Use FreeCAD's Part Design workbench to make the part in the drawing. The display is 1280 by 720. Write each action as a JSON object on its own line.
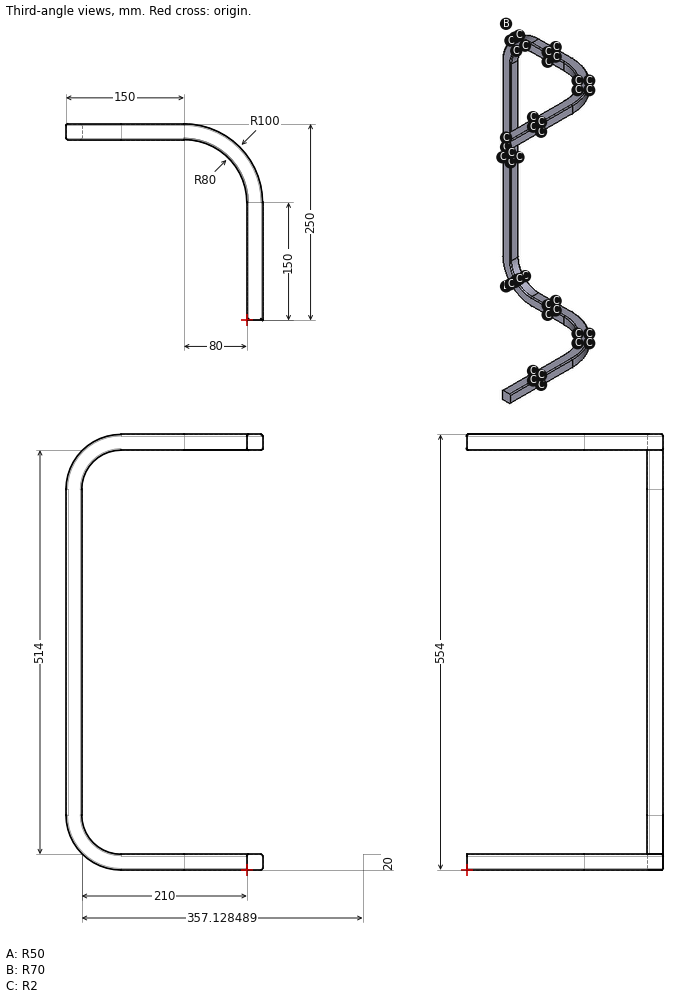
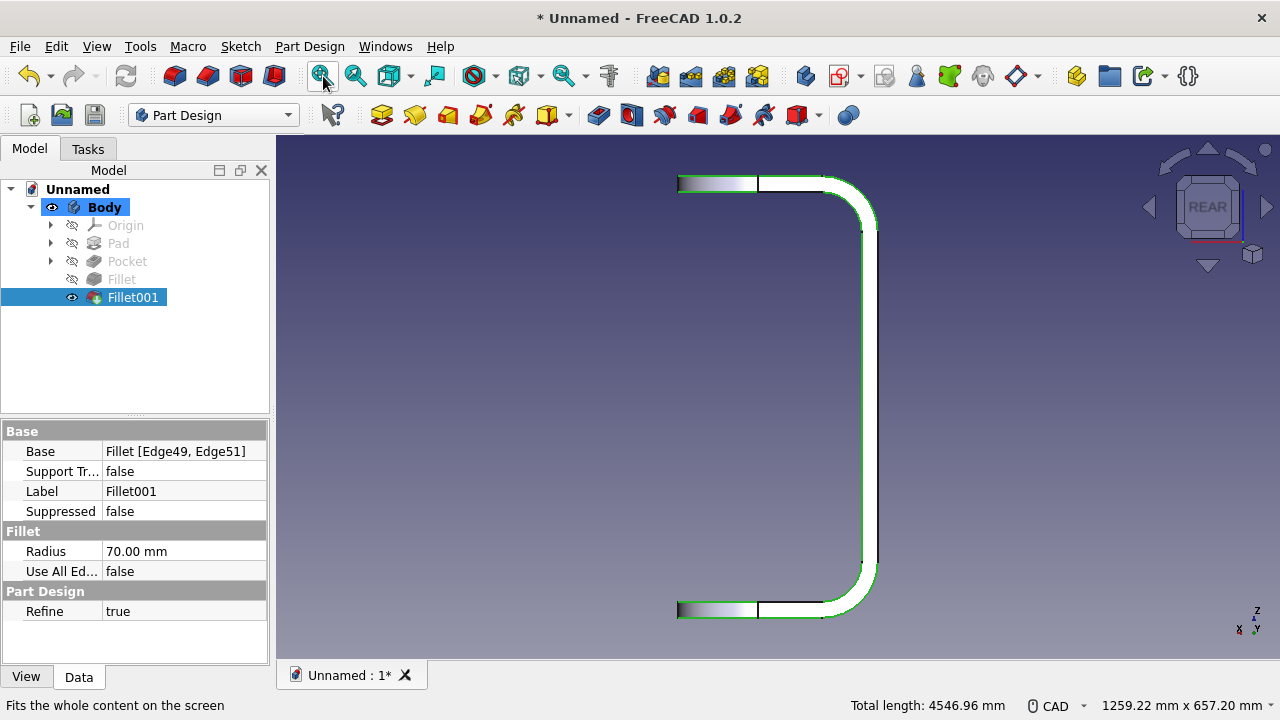
{"action": "left_click", "coordinate": [790, 601], "text": "ctrl"}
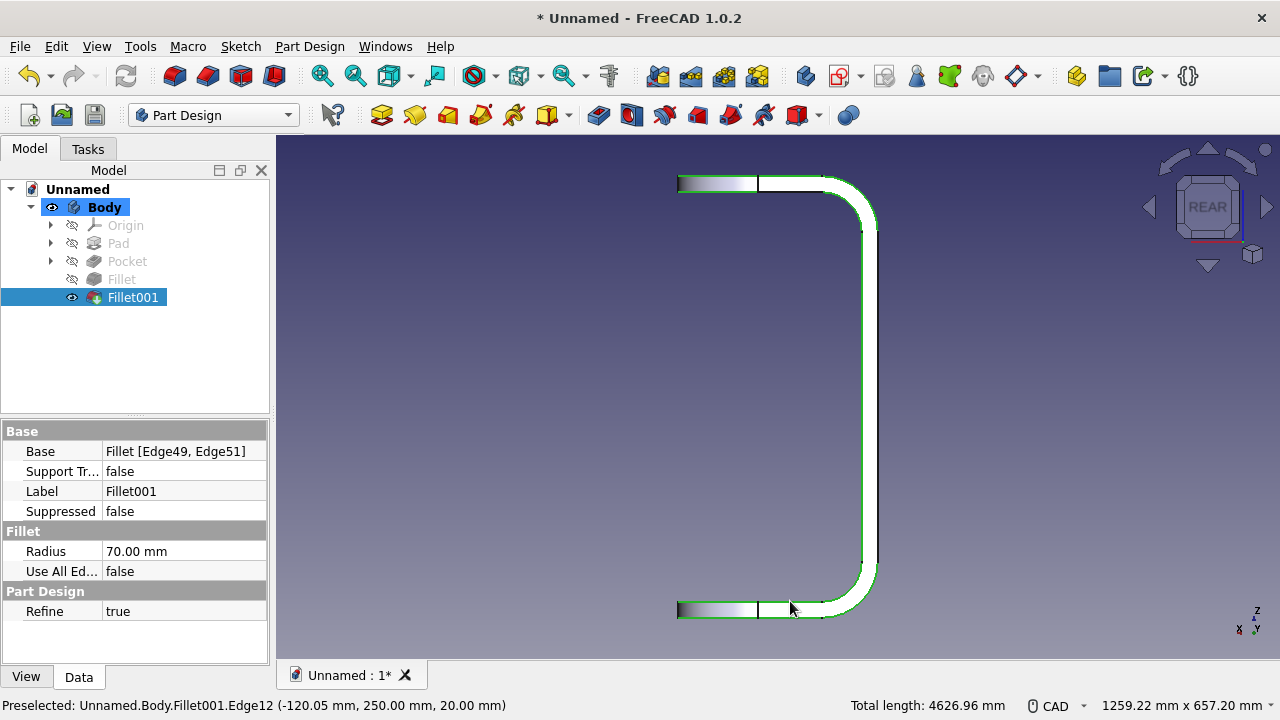
{"action": "left_click", "coordinate": [790, 191], "text": "ctrl"}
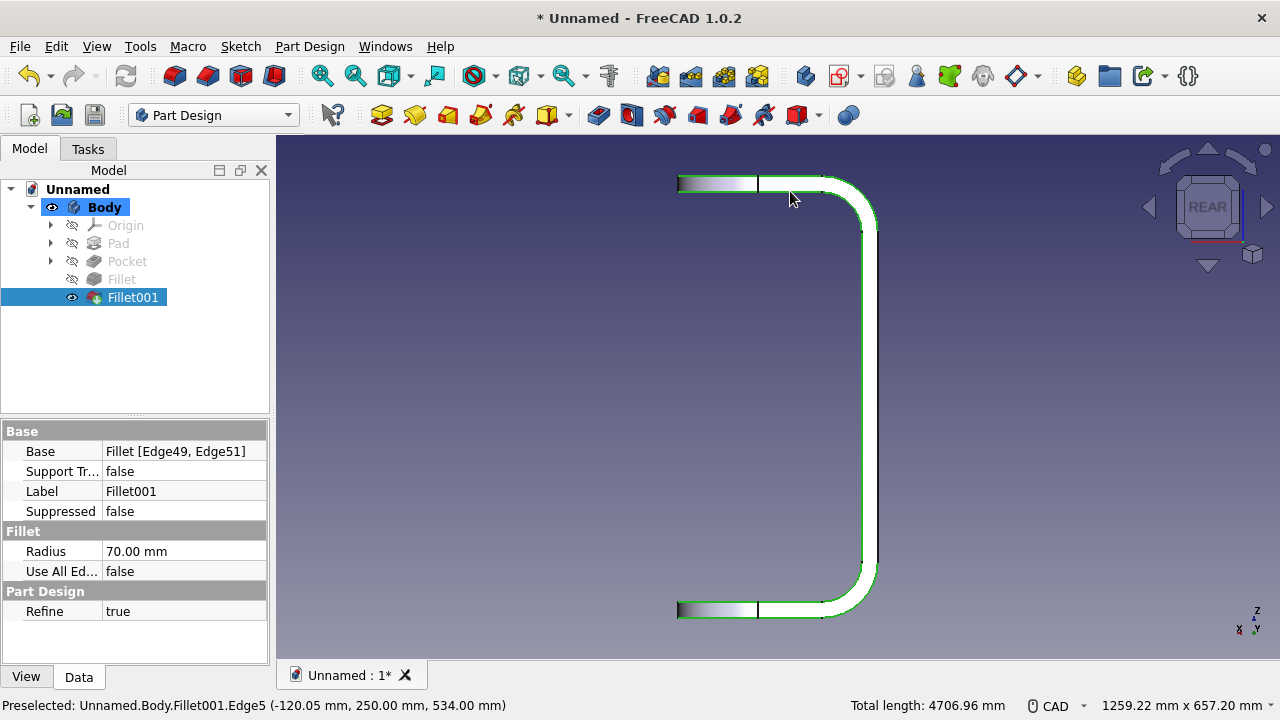
{"action": "left_click", "coordinate": [878, 396], "text": "ctrl"}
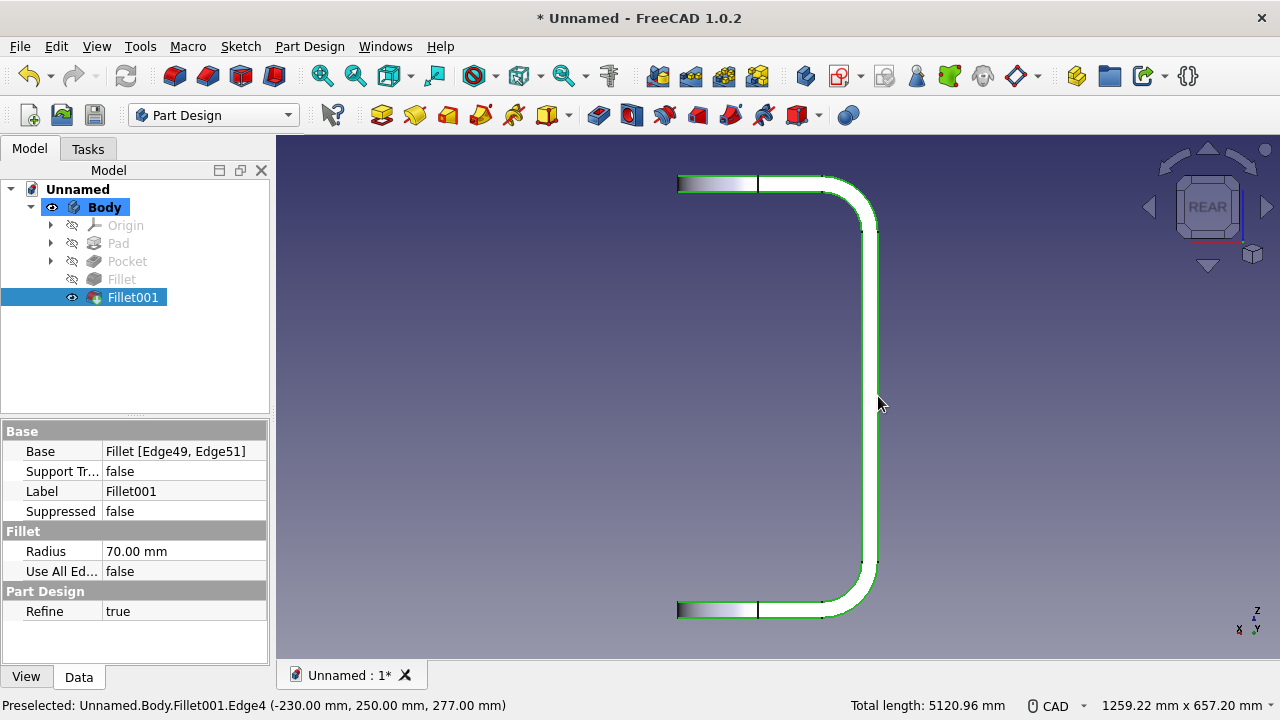
{"action": "key", "text": "6"}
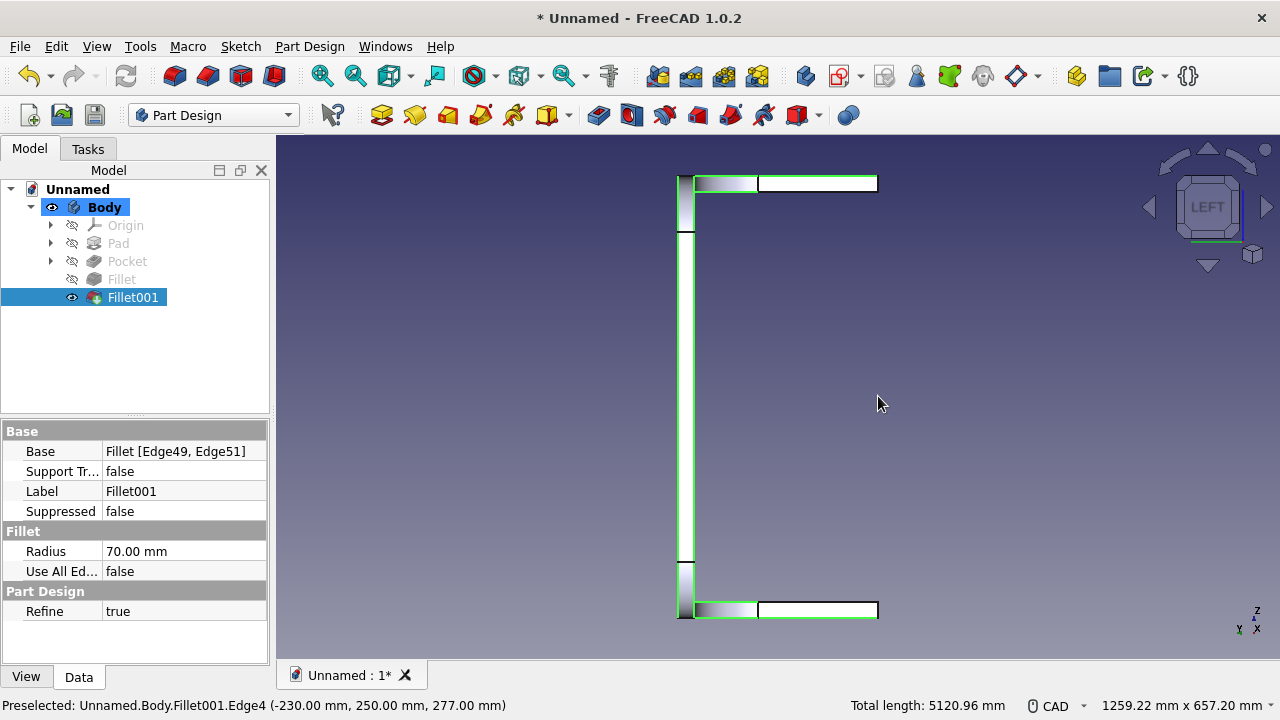
{"action": "left_click", "coordinate": [818, 191], "text": "ctrl"}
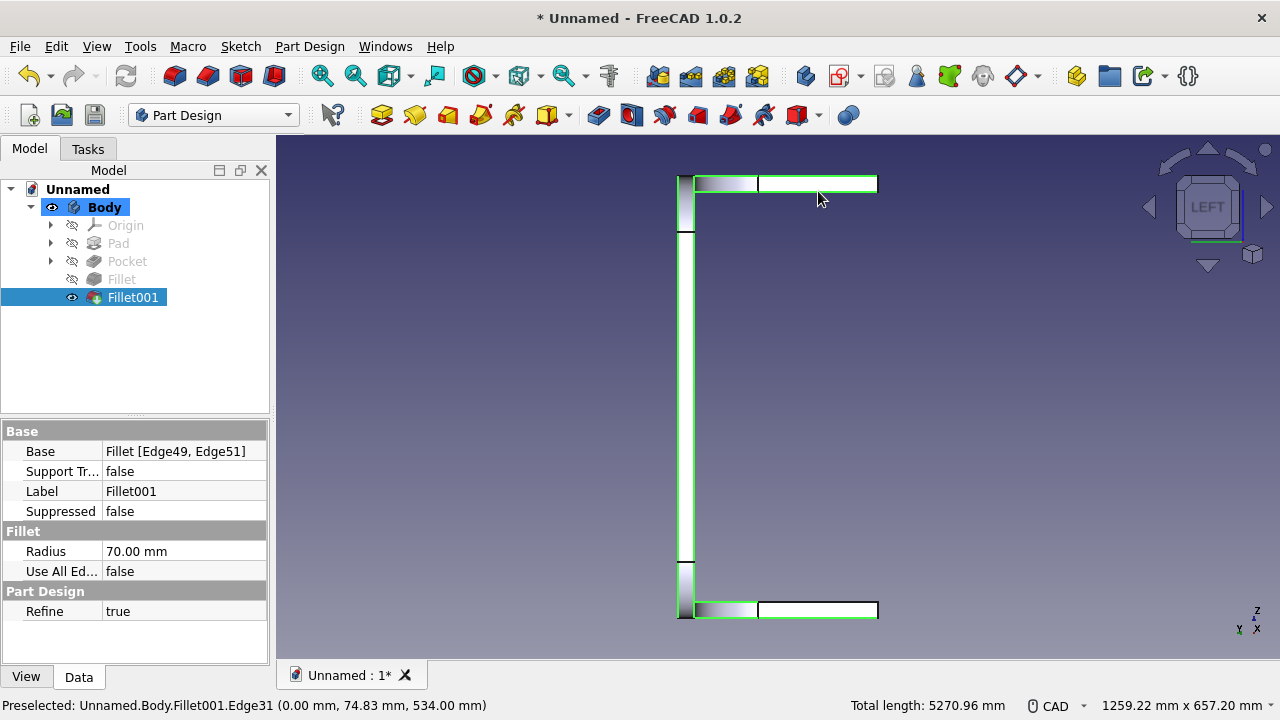
{"action": "left_click", "coordinate": [818, 601], "text": "ctrl"}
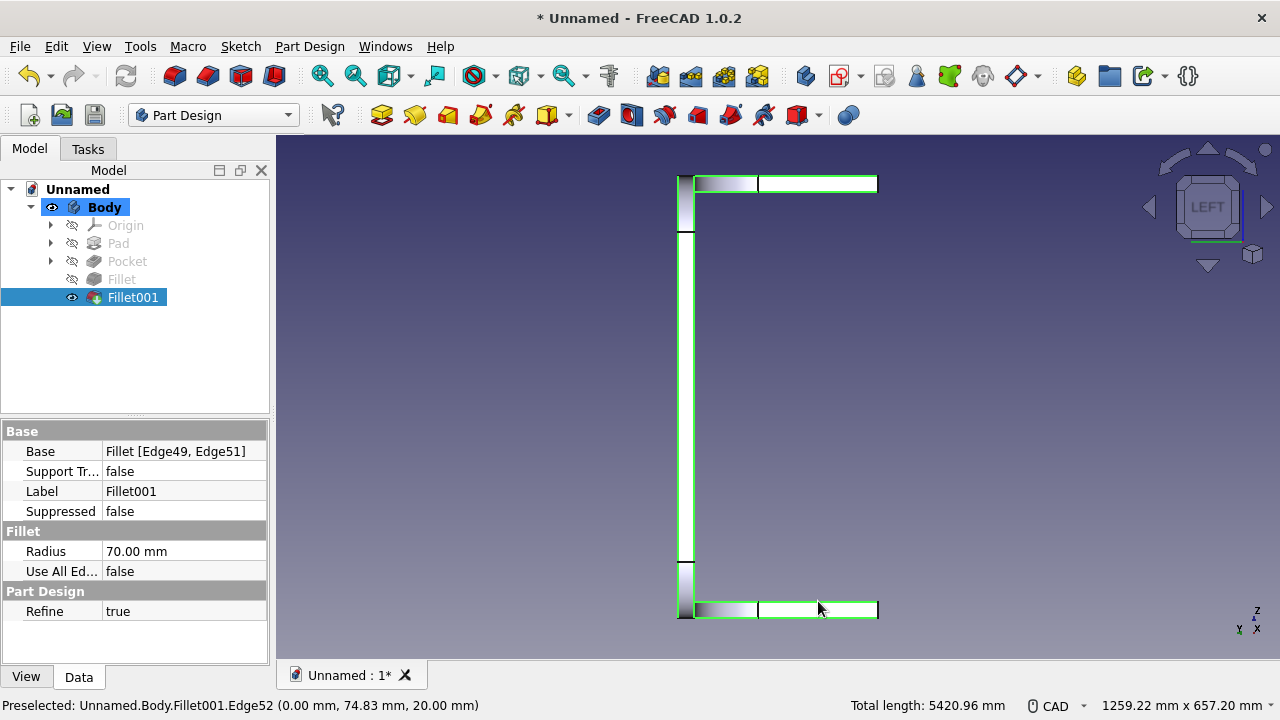
{"action": "left_click", "coordinate": [175, 76]}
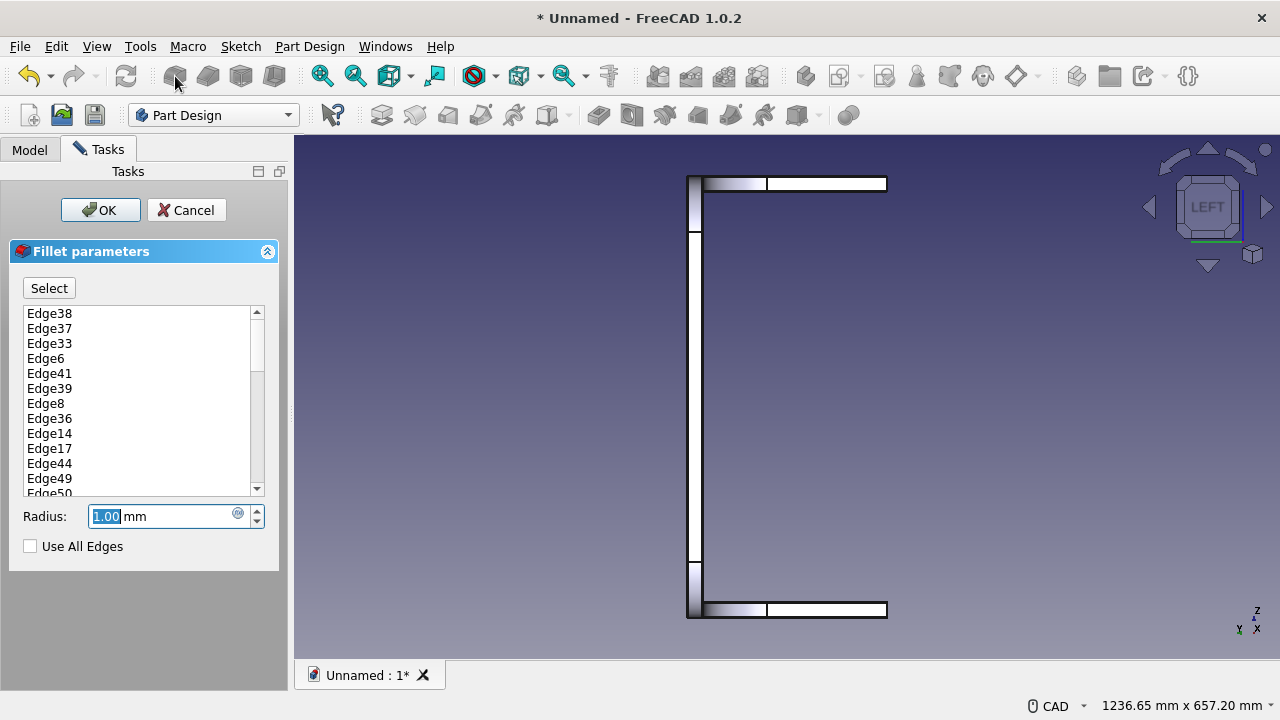
{"action": "type", "text": "2"}
{"action": "key", "text": "Tab"}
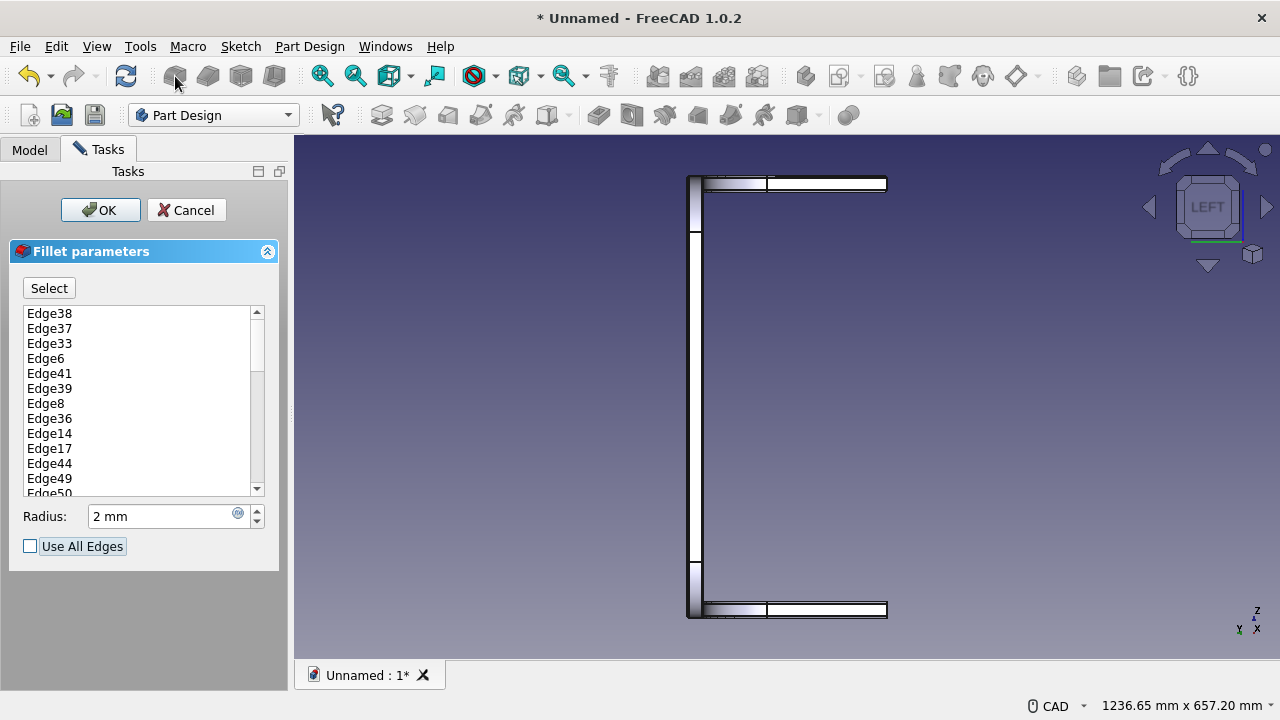
{"action": "left_click", "coordinate": [101, 210]}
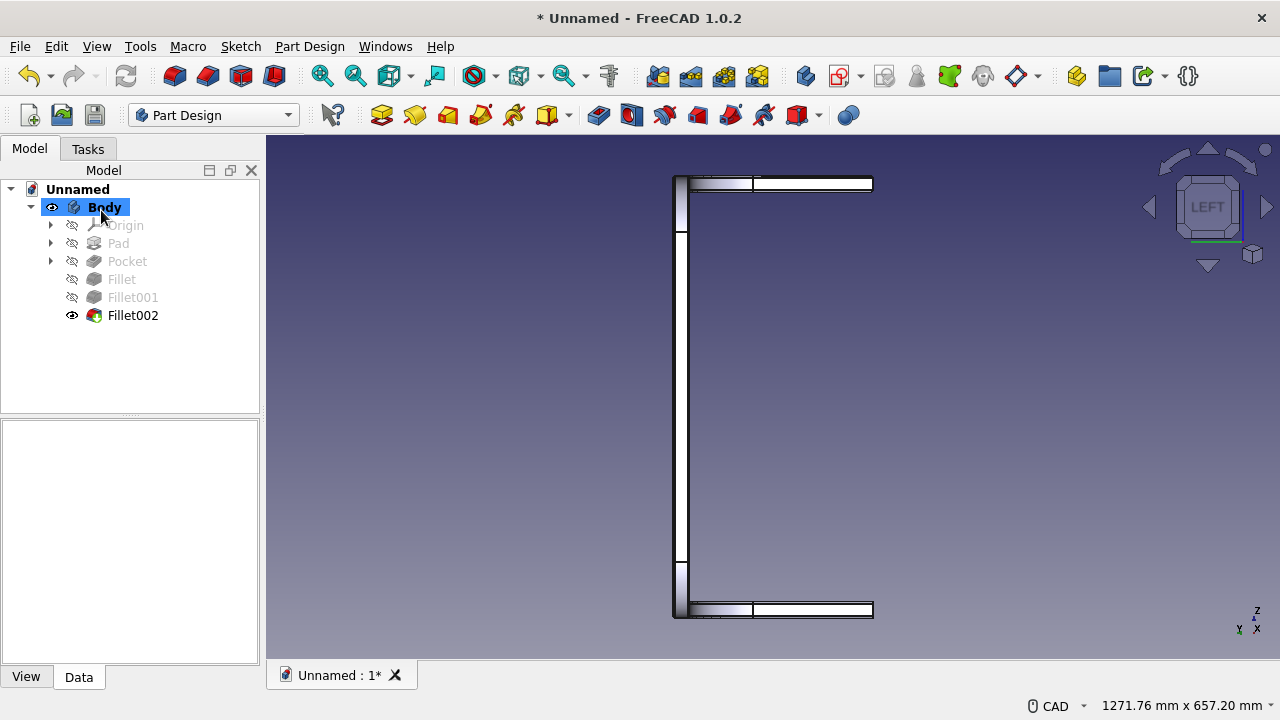
{"action": "key", "text": "0"}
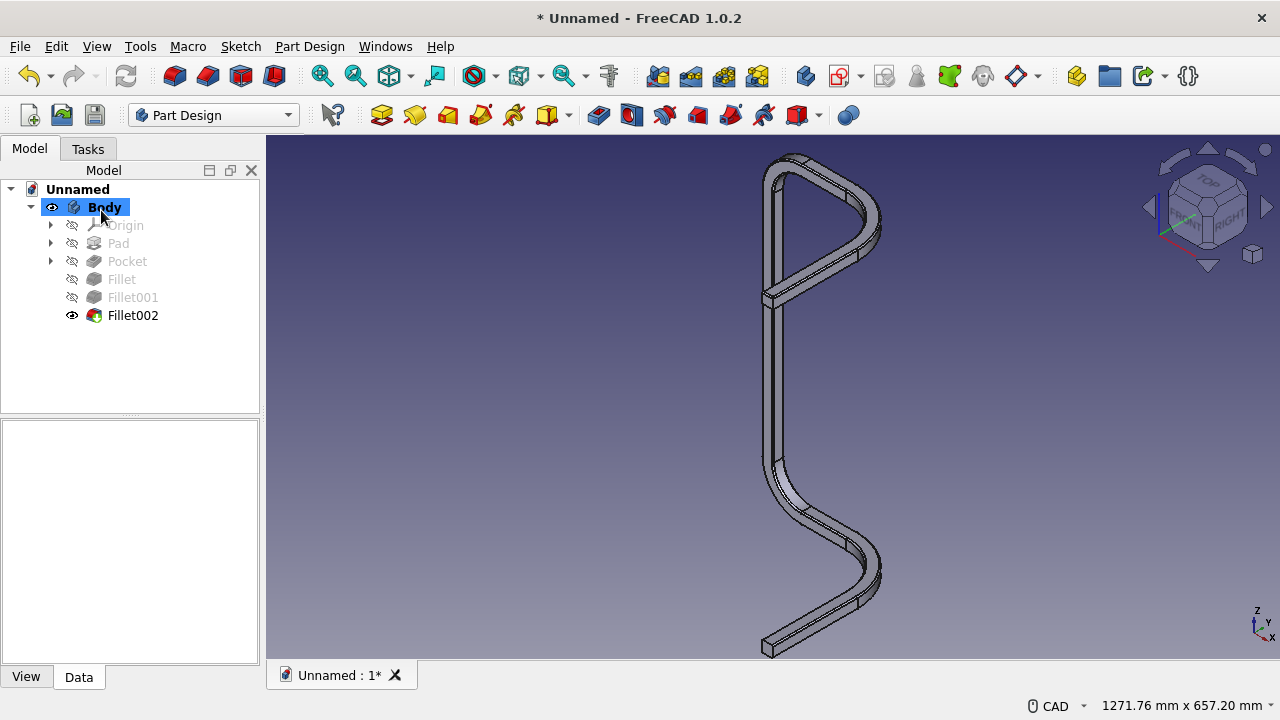
{"action": "left_click", "coordinate": [323, 76]}